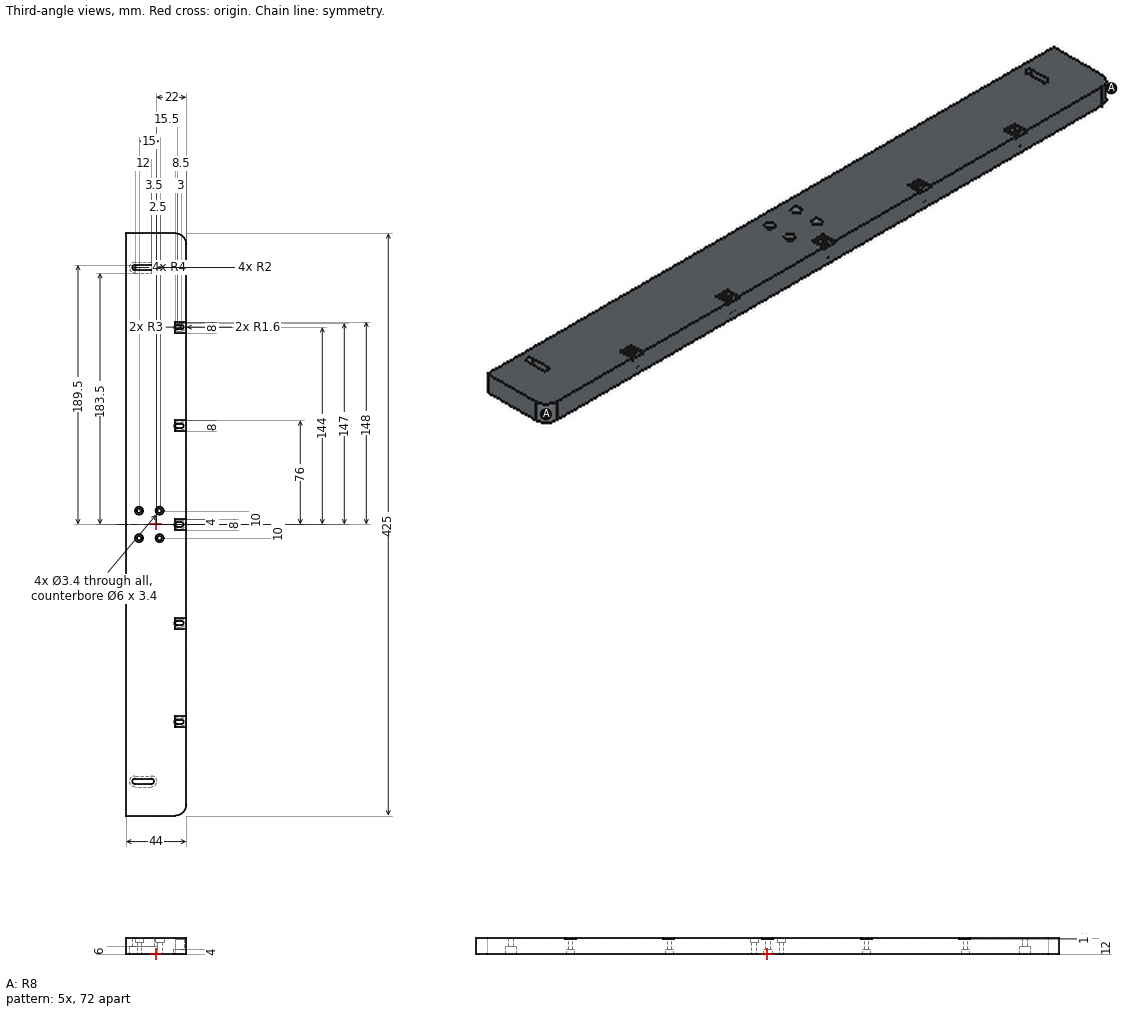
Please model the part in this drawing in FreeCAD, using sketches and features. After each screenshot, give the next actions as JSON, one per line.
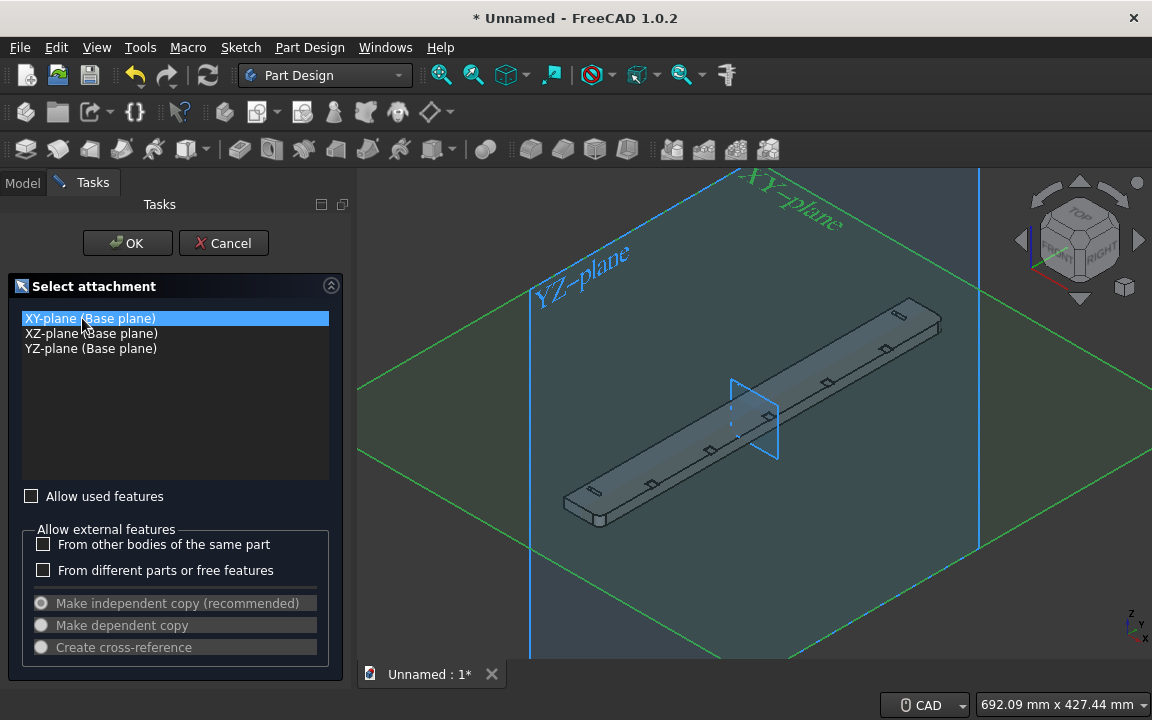
{"action": "left_click", "coordinate": [128, 243]}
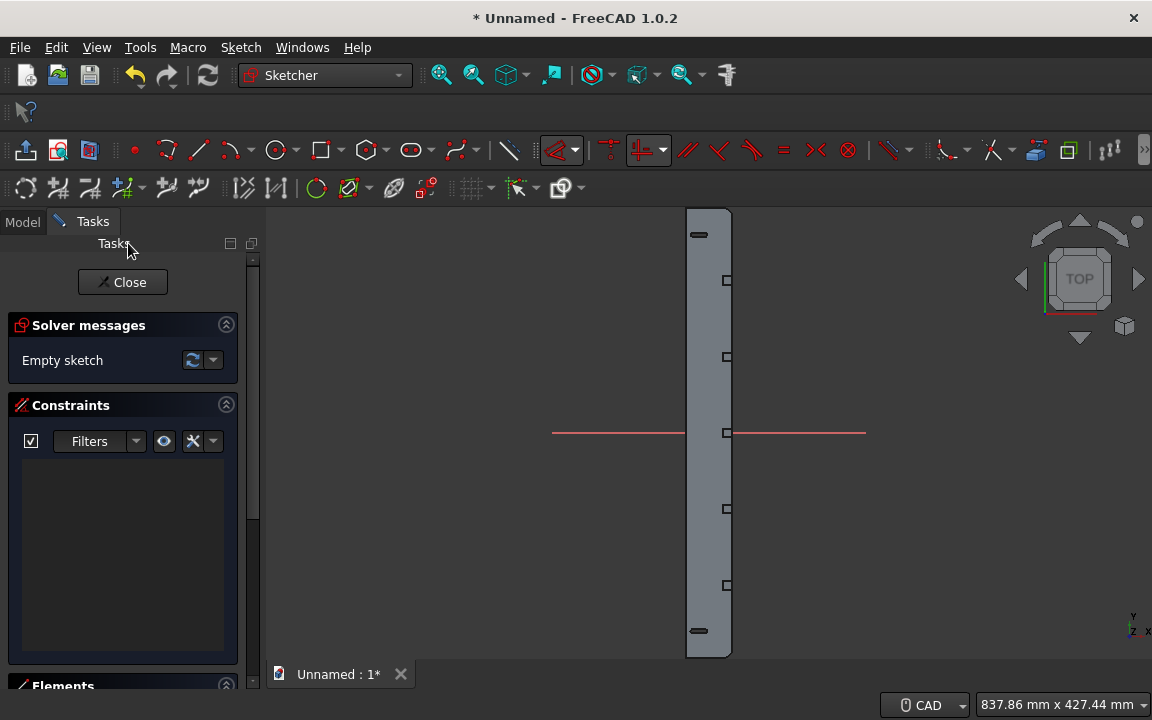
{"action": "key", "text": "q s"}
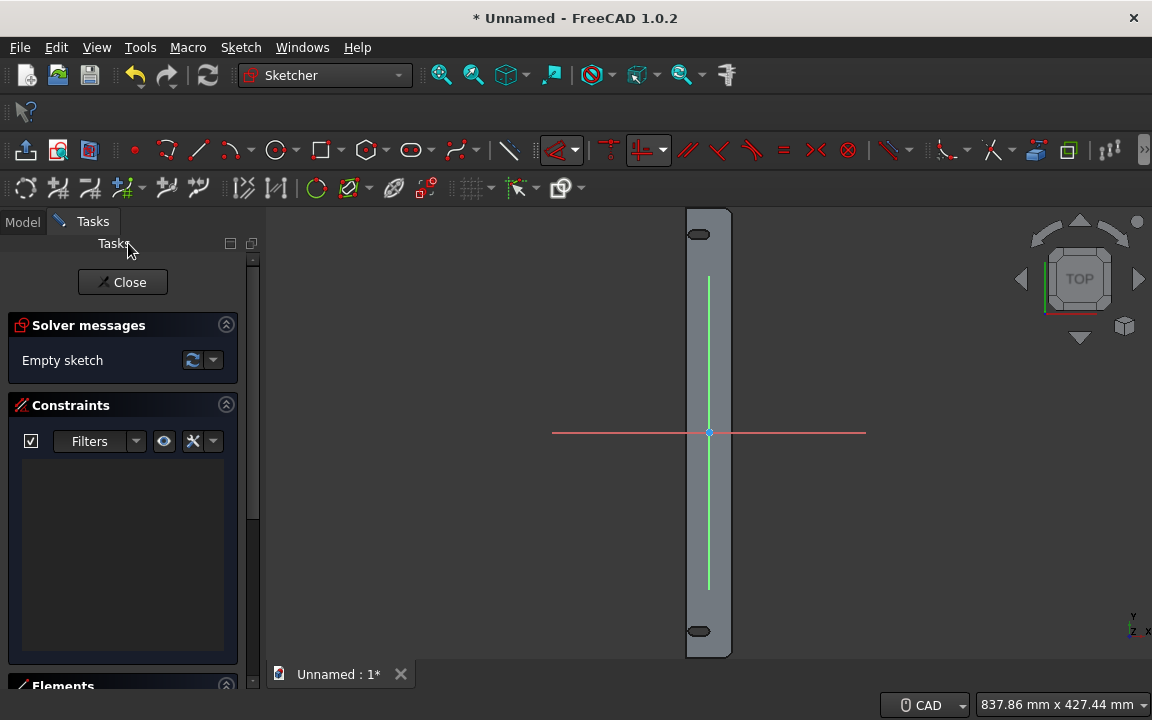
{"action": "scroll", "coordinate": [732, 273], "scroll_direction": "up", "scroll_amount": 15}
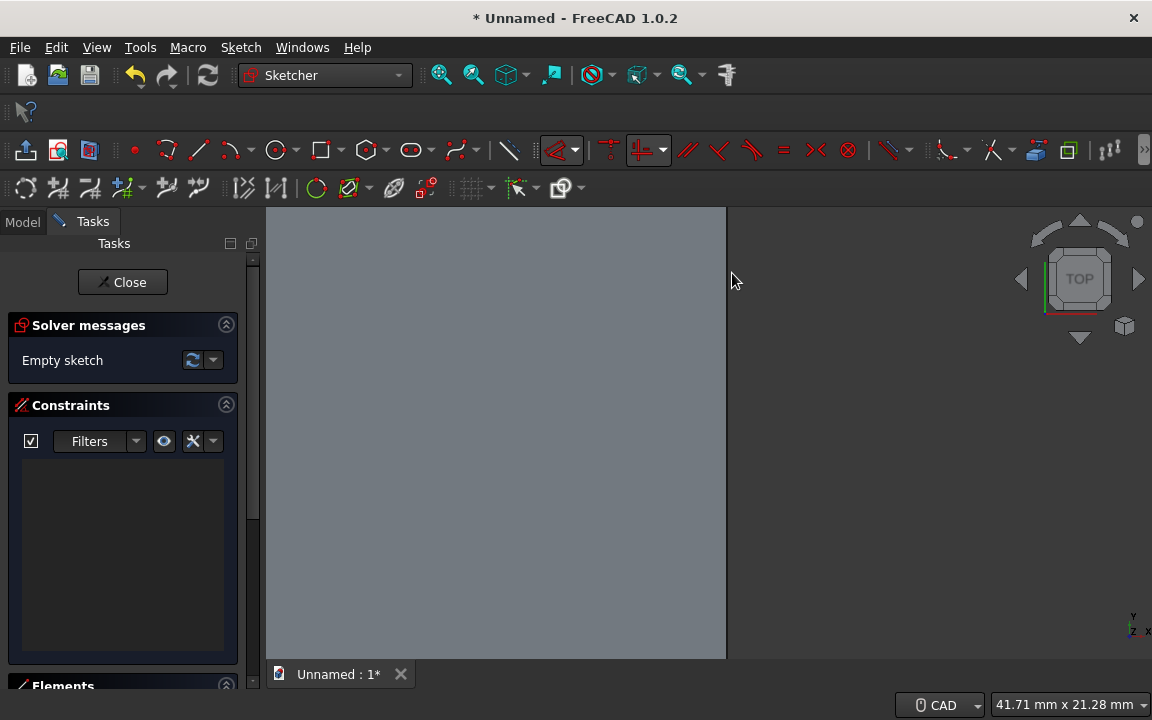
{"action": "scroll", "coordinate": [605, 419], "scroll_direction": "up", "scroll_amount": 4}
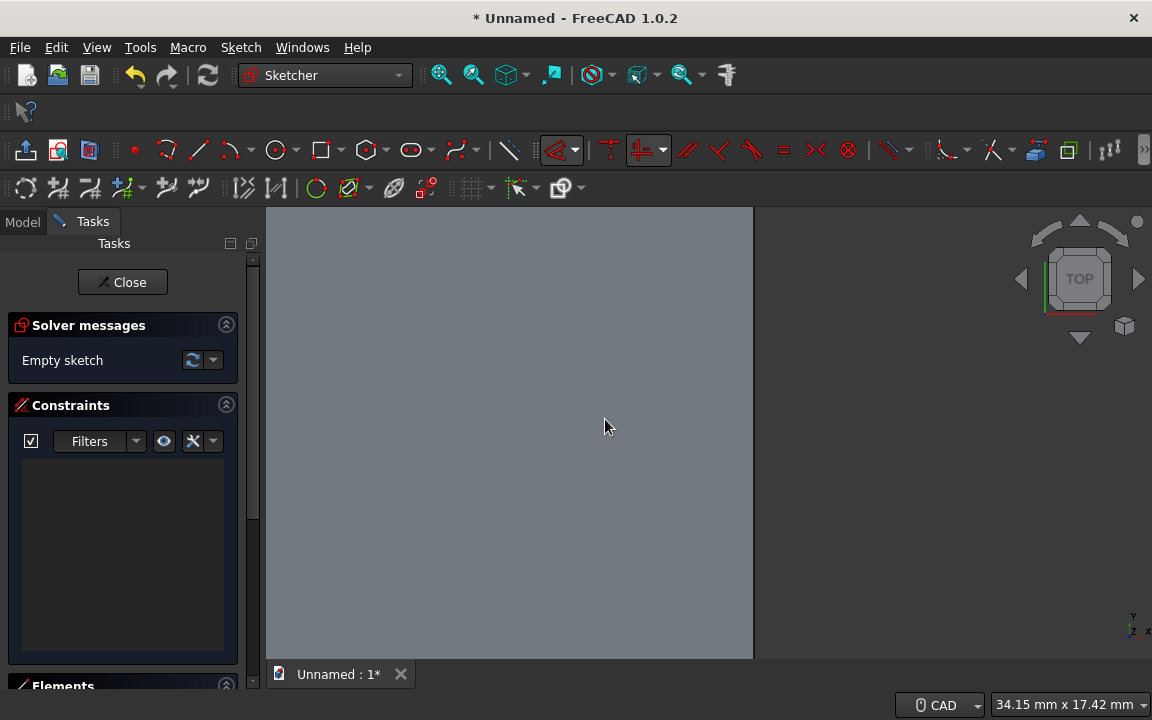
{"action": "key", "text": "g s"}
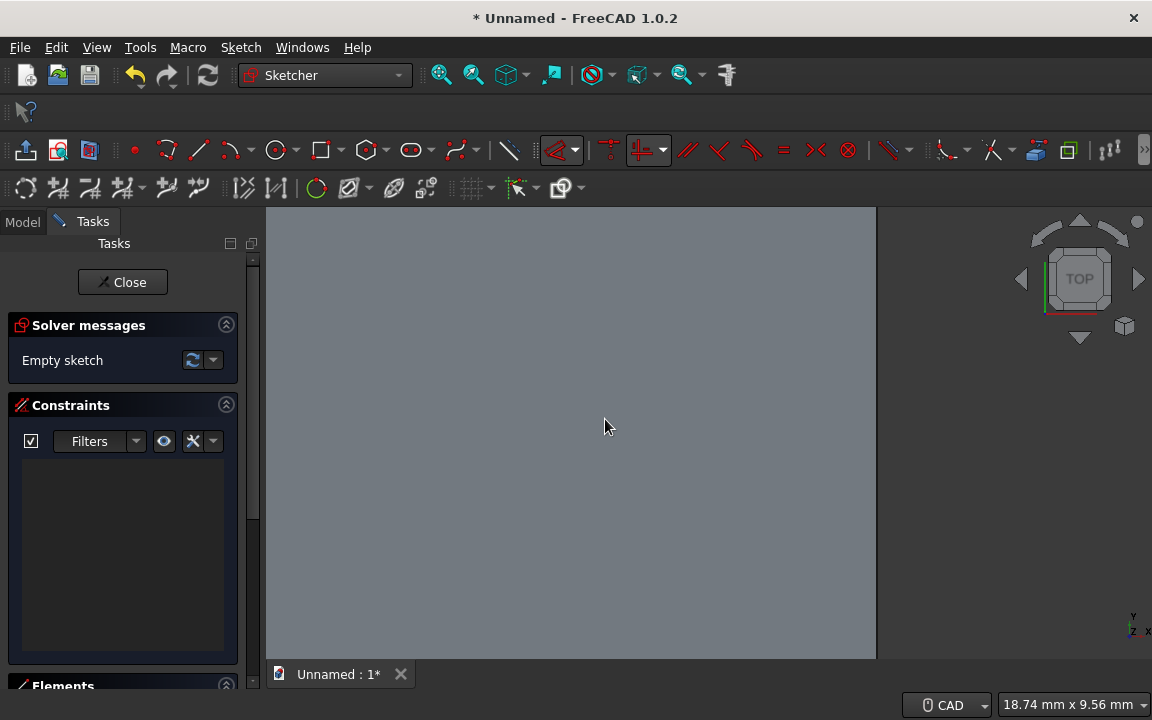
{"action": "left_click", "coordinate": [569, 433]}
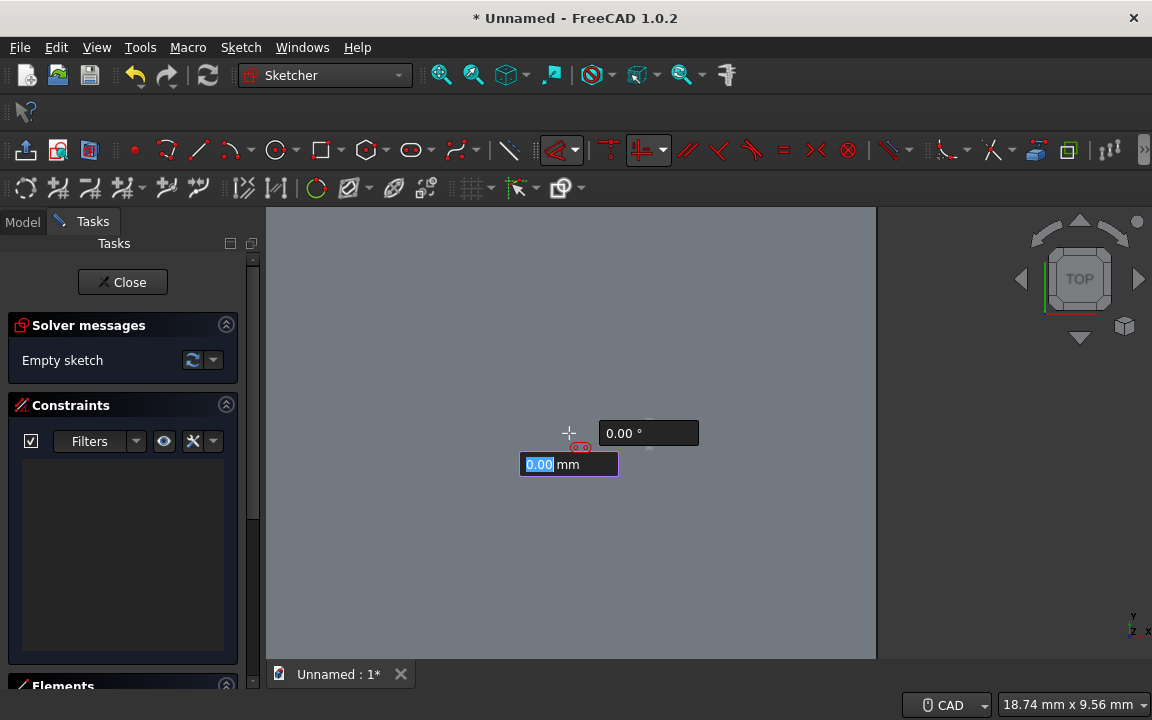
{"action": "left_click", "coordinate": [711, 433]}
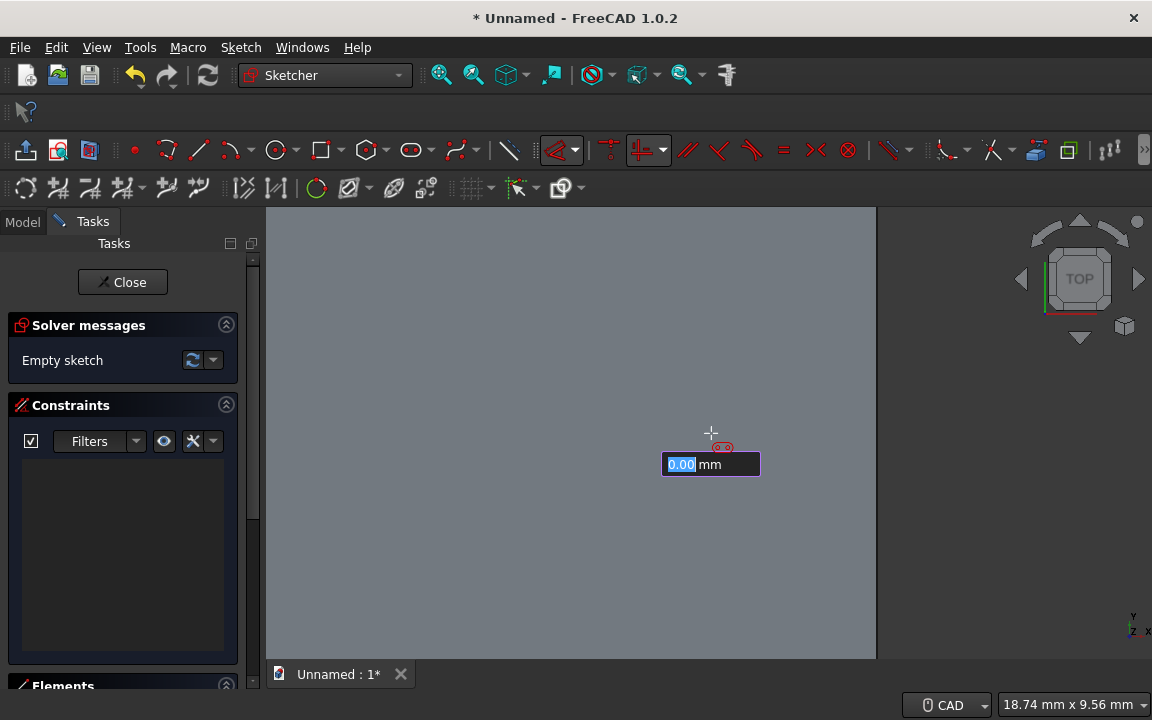
{"action": "left_click", "coordinate": [640, 291]}
{"action": "key", "text": "Escape"}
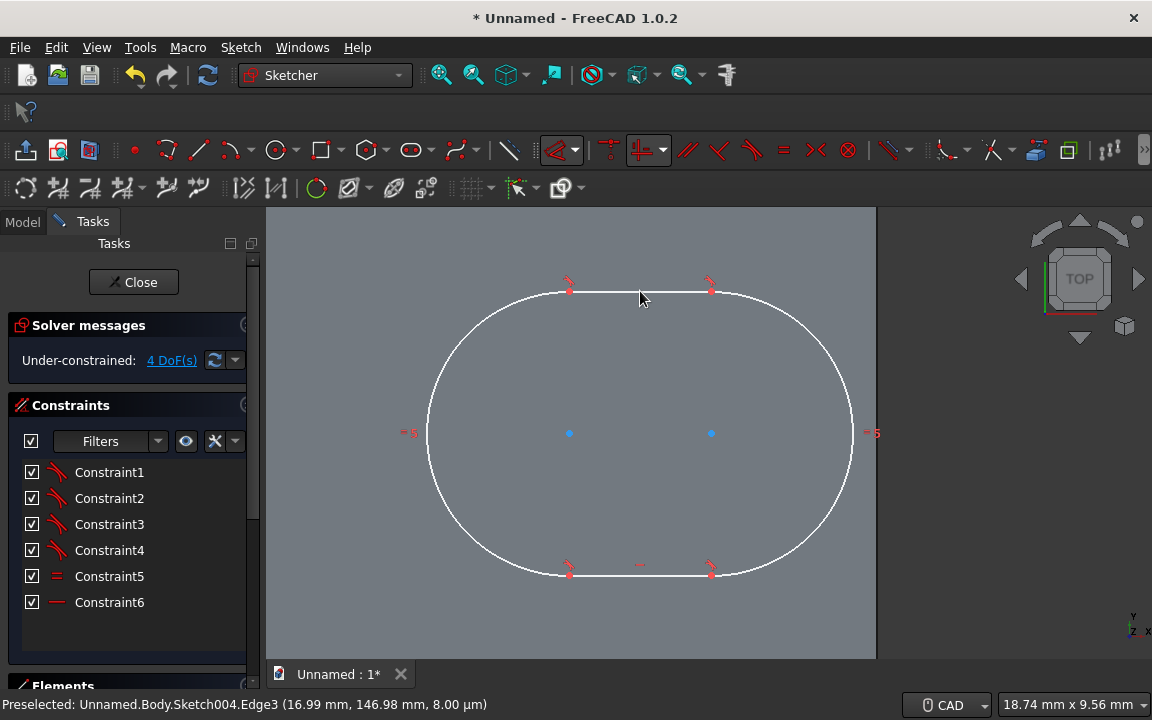
{"action": "left_click", "coordinate": [454, 351]}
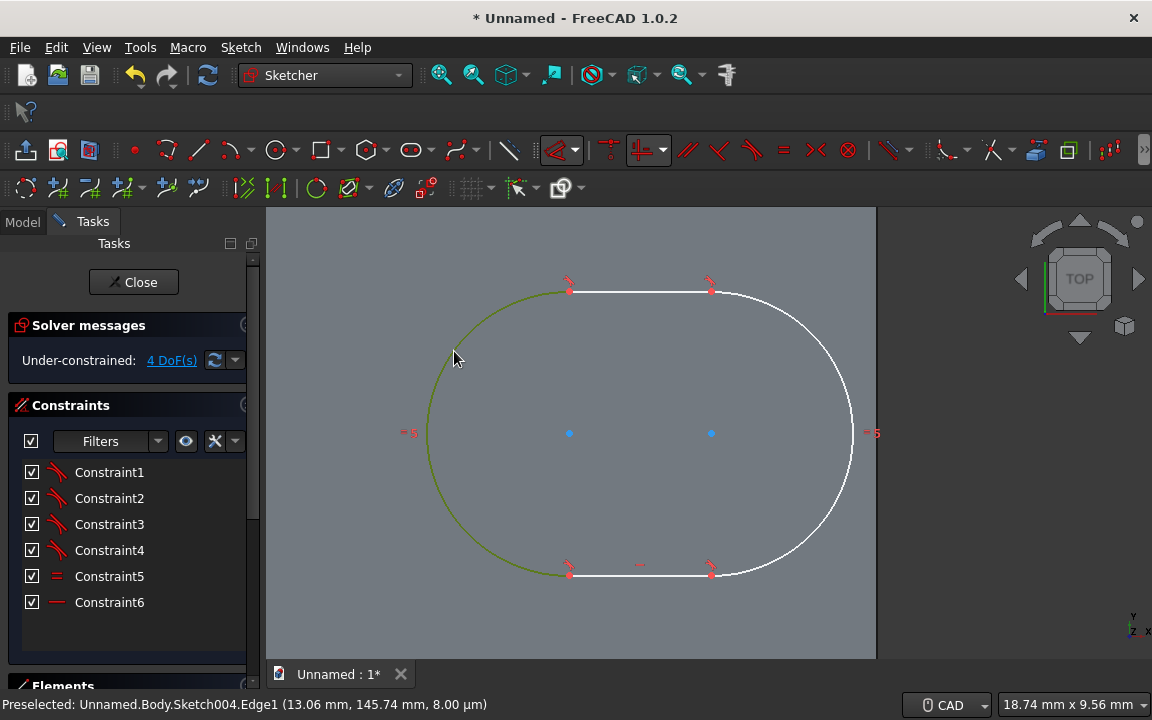
{"action": "left_click", "coordinate": [578, 150]}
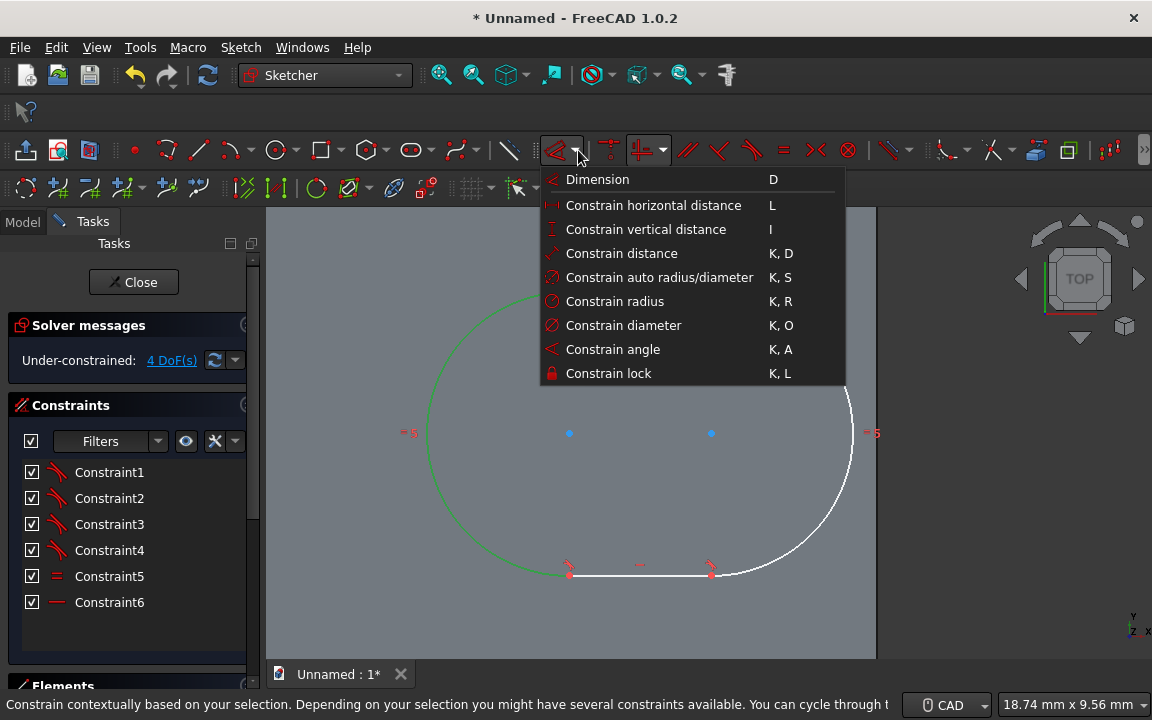
{"action": "left_click", "coordinate": [693, 301]}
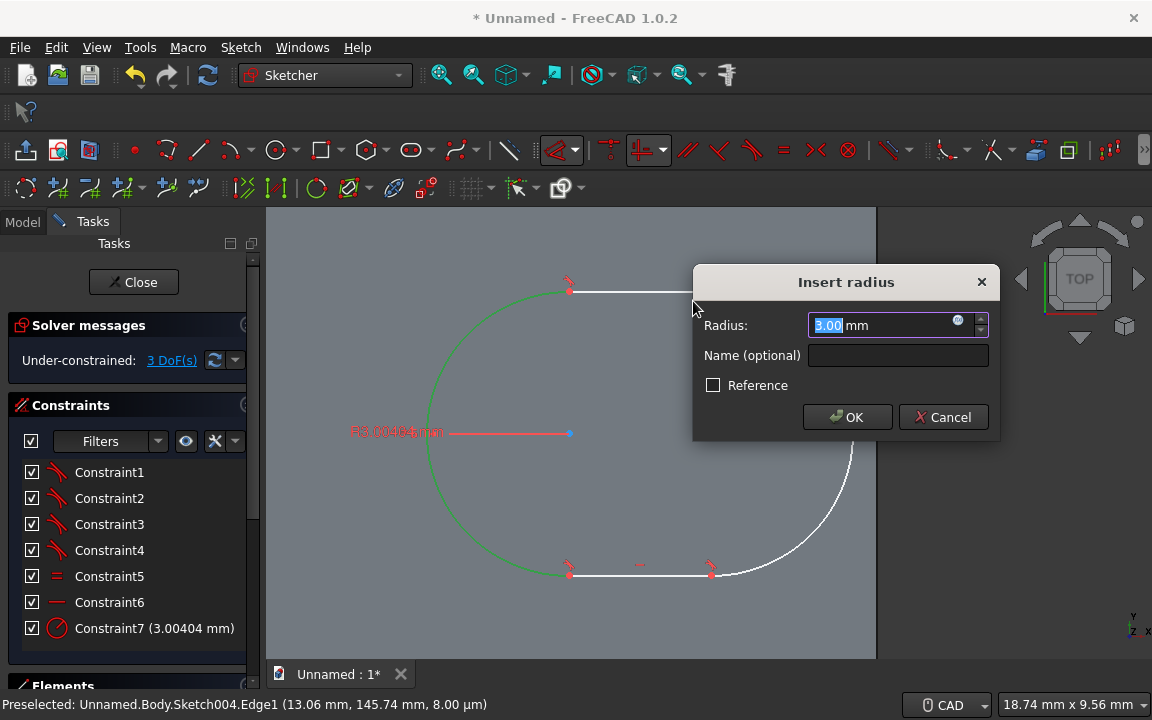
{"action": "type", "text": "3"}
{"action": "key", "text": "Return"}